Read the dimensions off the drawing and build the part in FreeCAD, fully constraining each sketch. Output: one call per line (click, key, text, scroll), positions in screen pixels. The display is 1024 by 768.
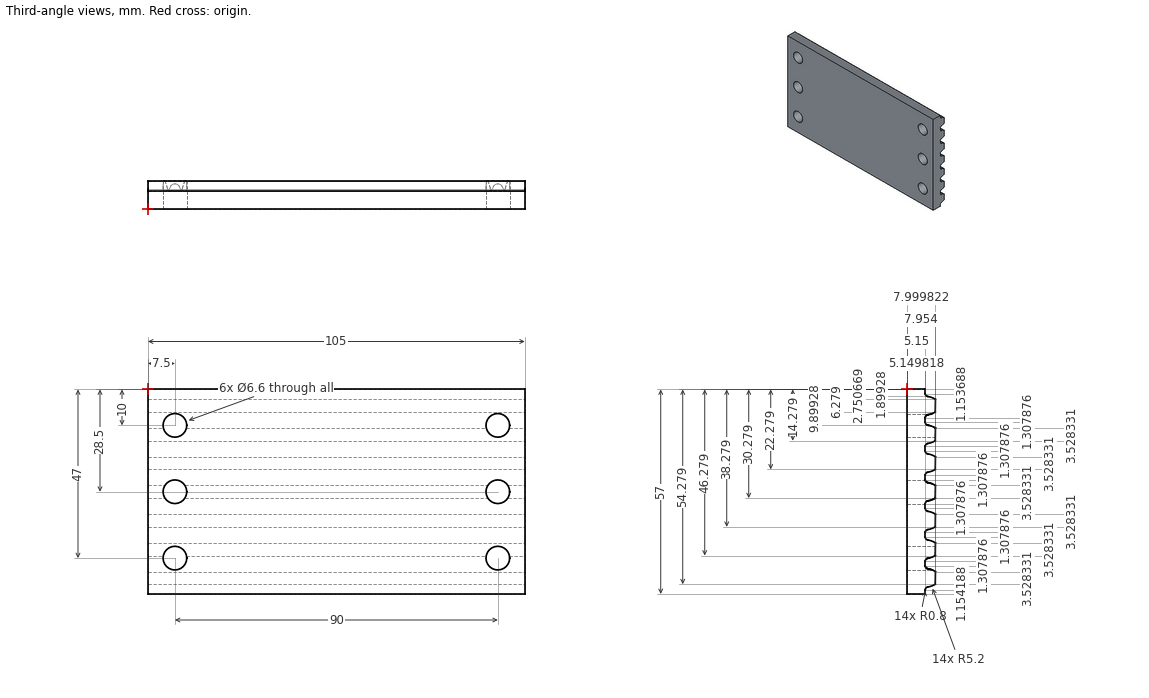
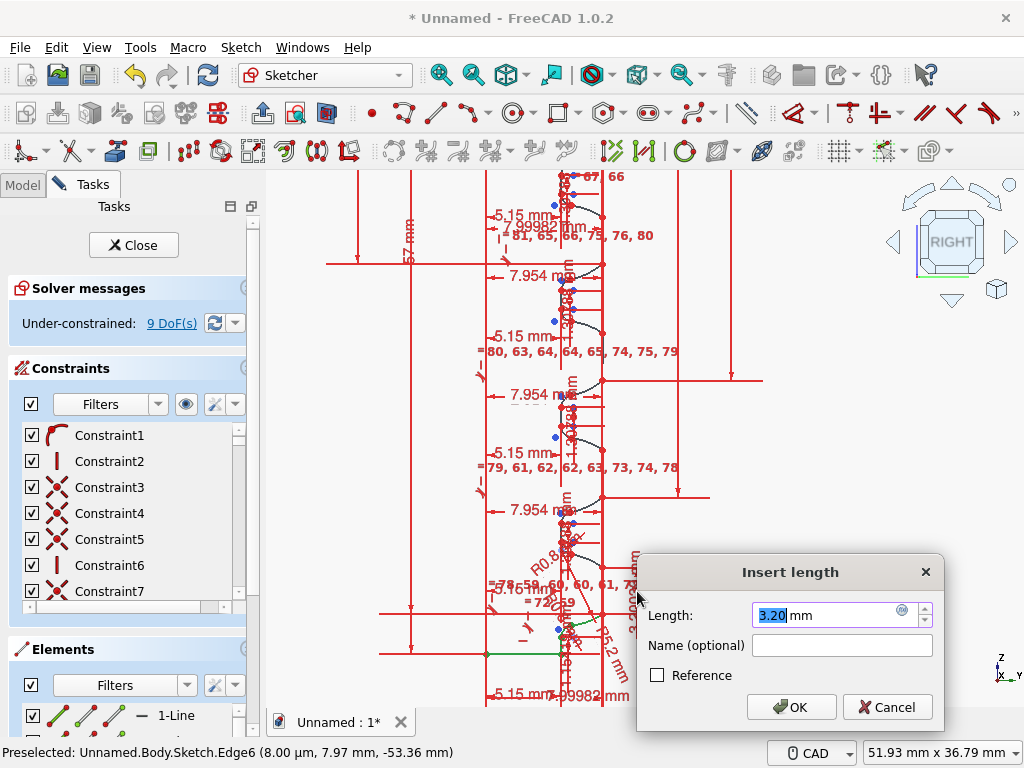
text(3.528331)
key(Return)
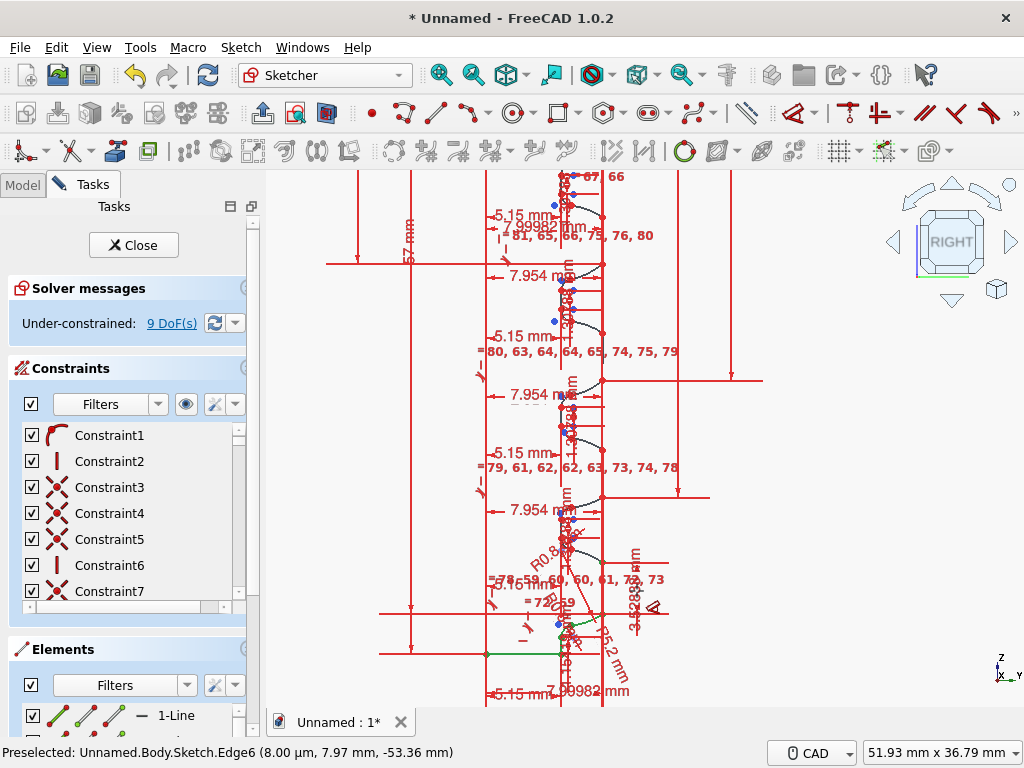
click(602, 483)
click(637, 474)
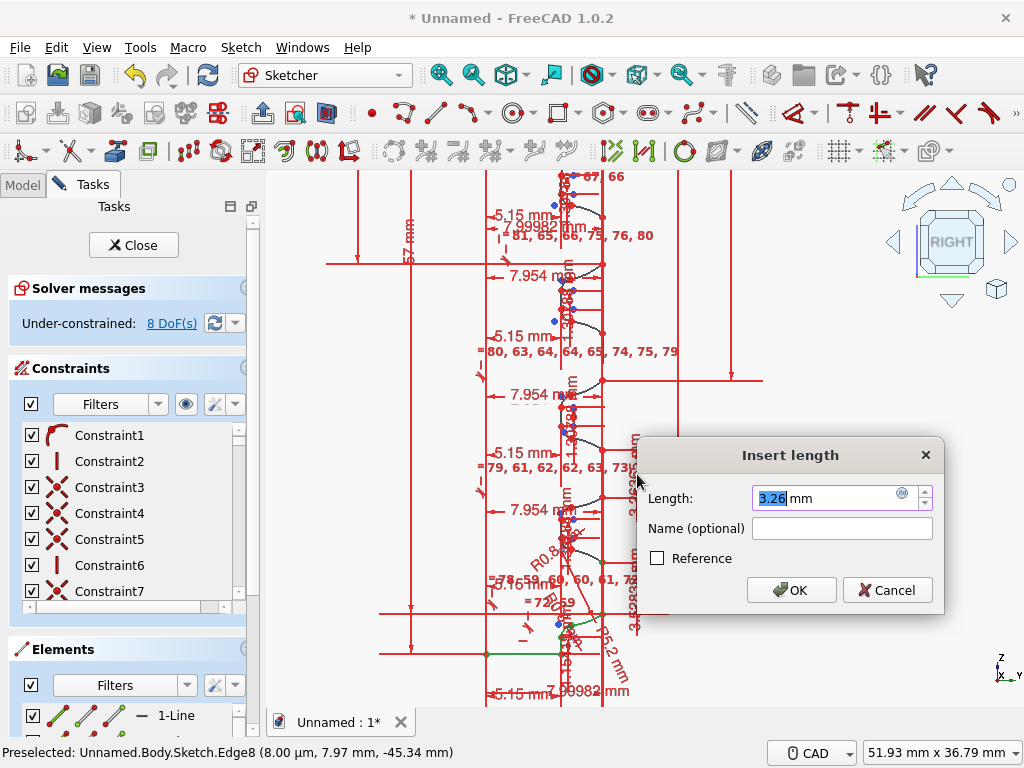
text(3.528331)
key(Return)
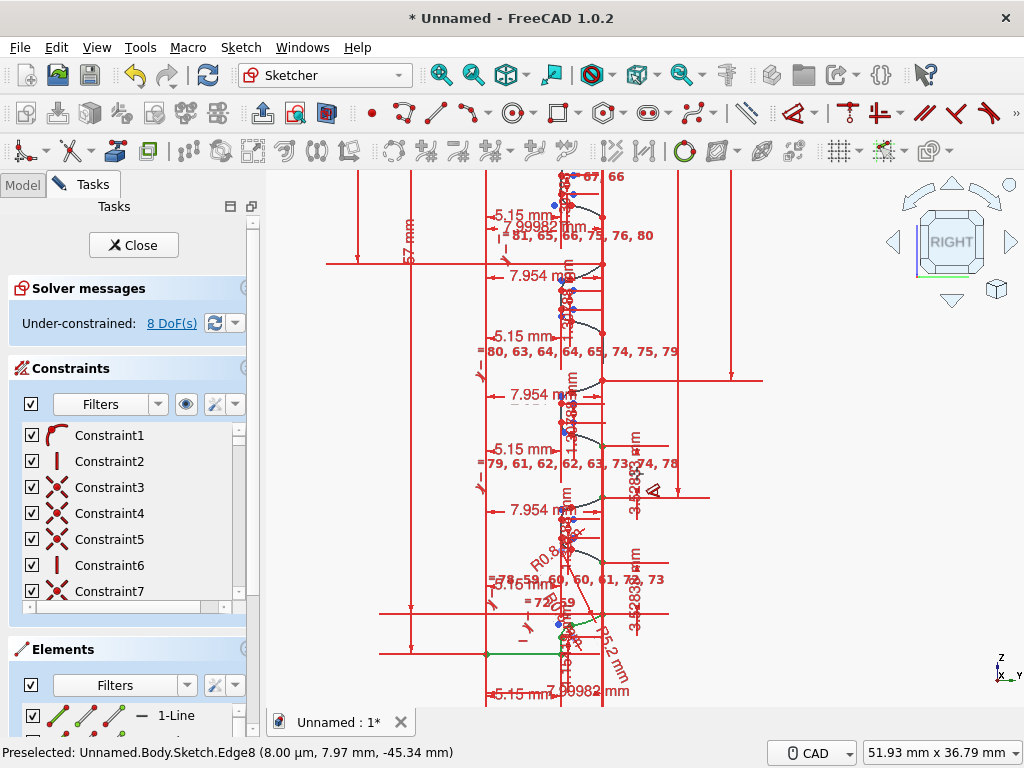
click(602, 367)
click(637, 357)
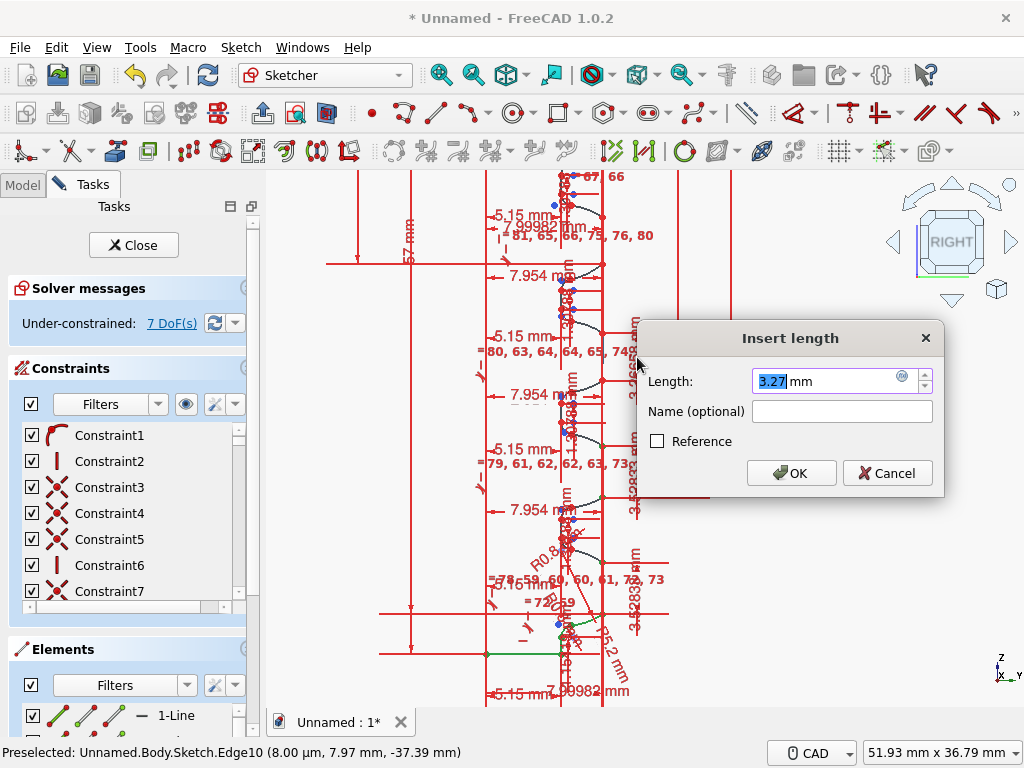
text(3.528331)
key(Return)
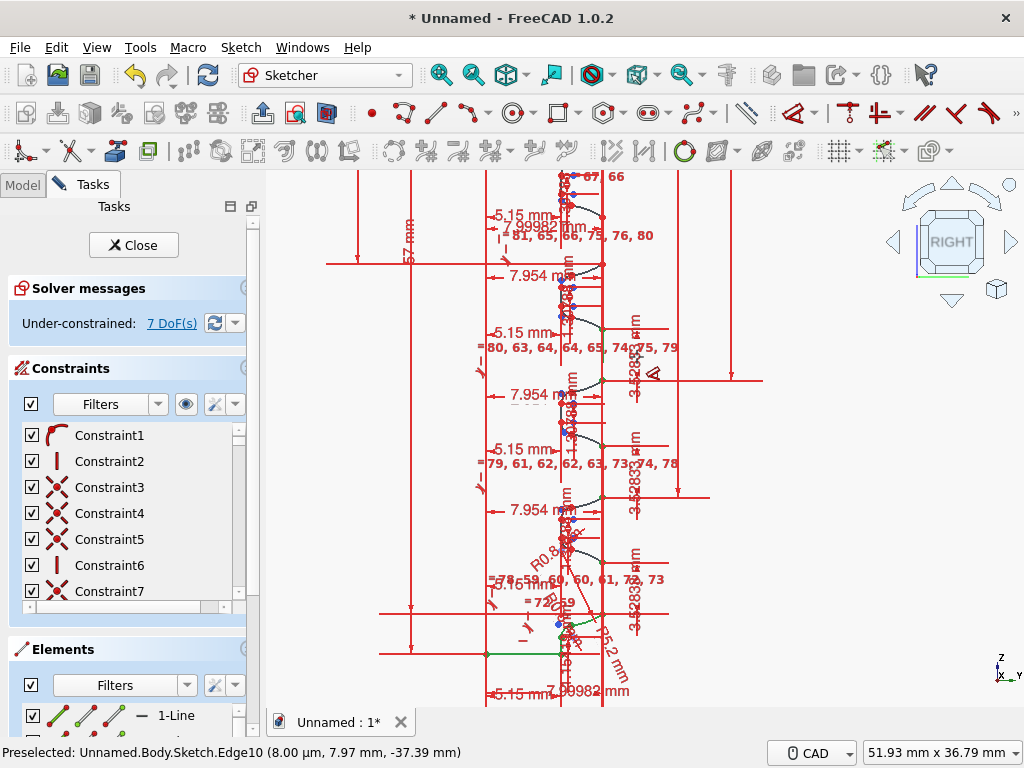
click(602, 250)
click(637, 241)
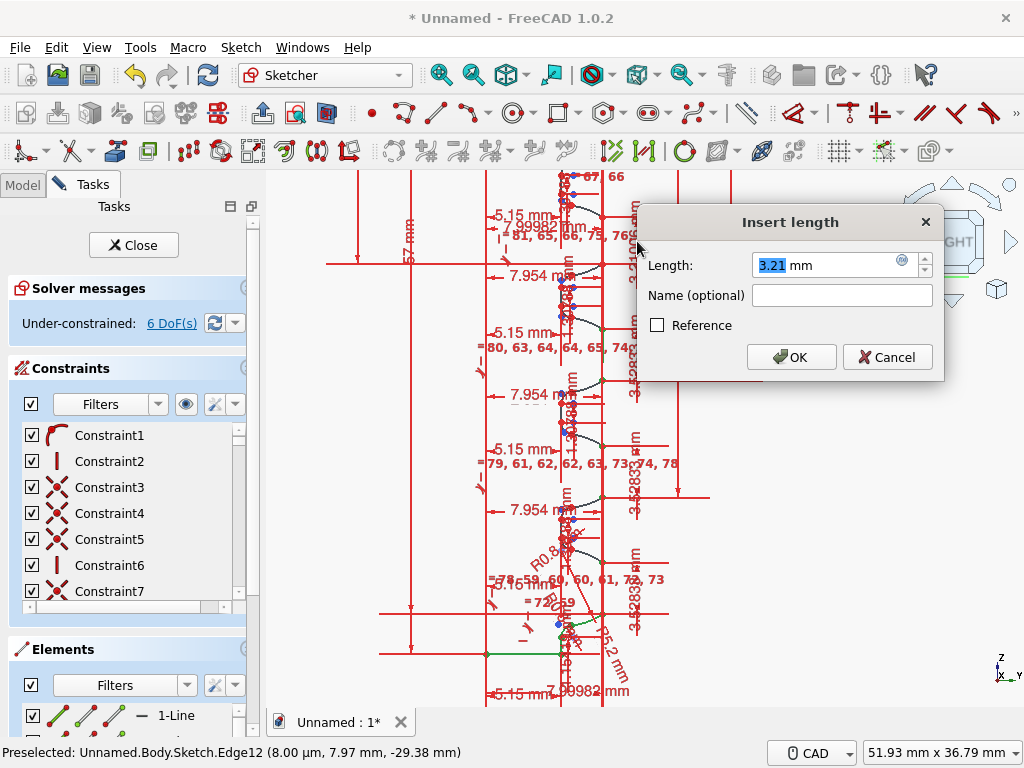
text(3.528331)
key(Return)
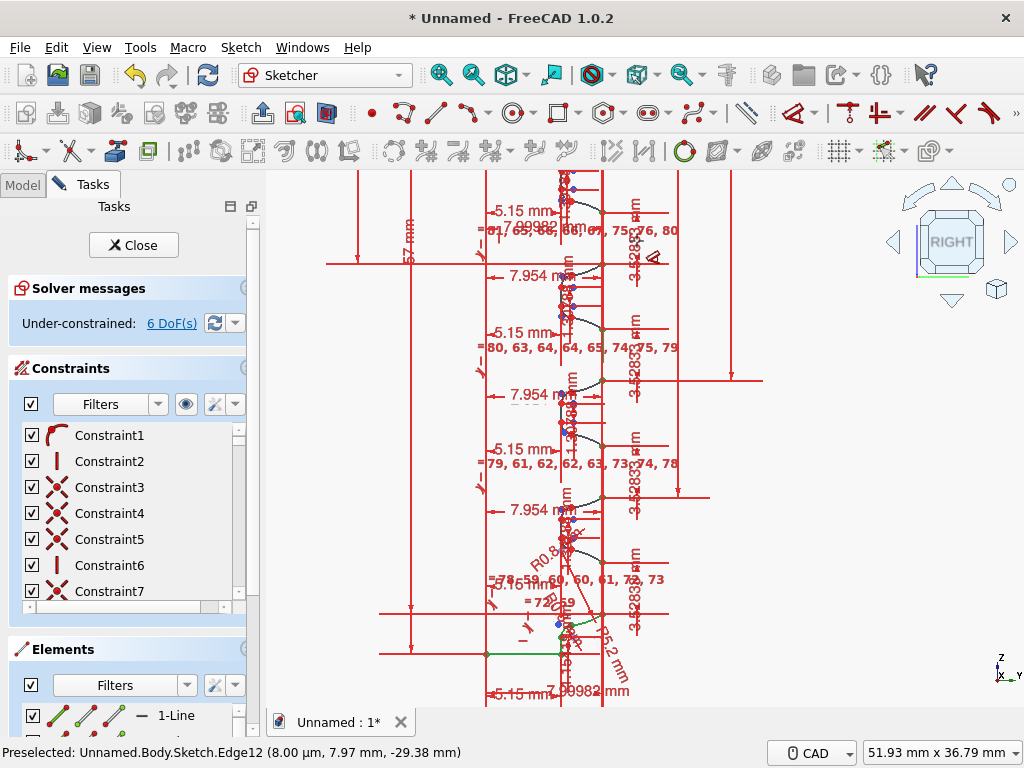
scroll(603, 602, down, 4)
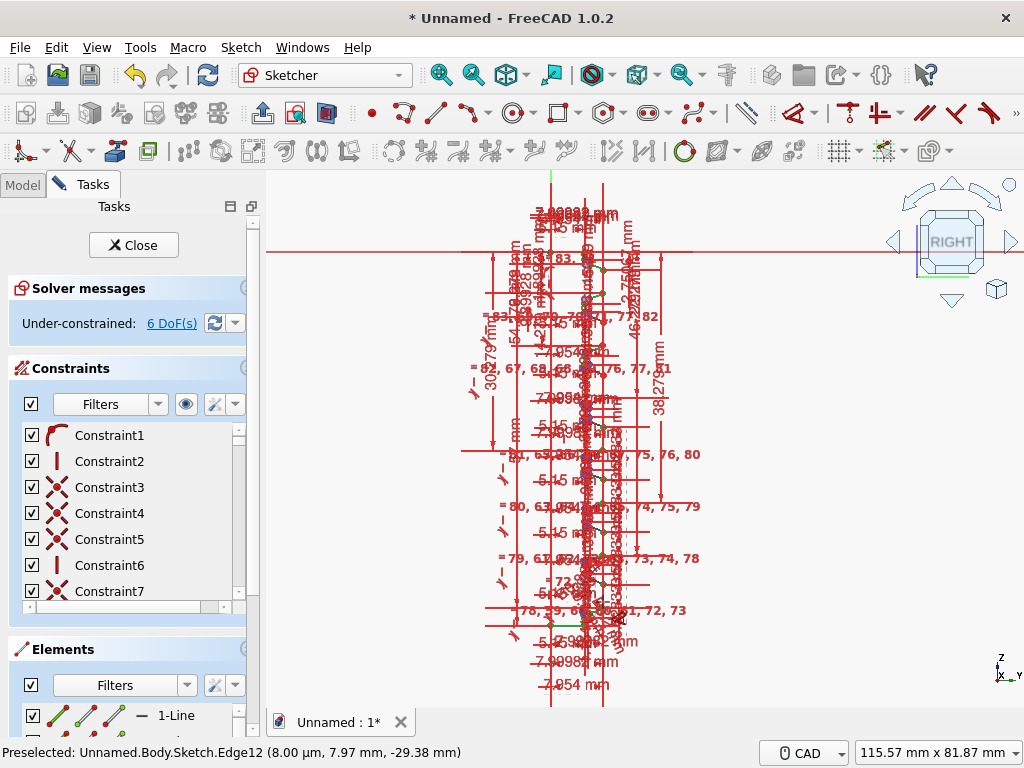
scroll(603, 391, up, 4)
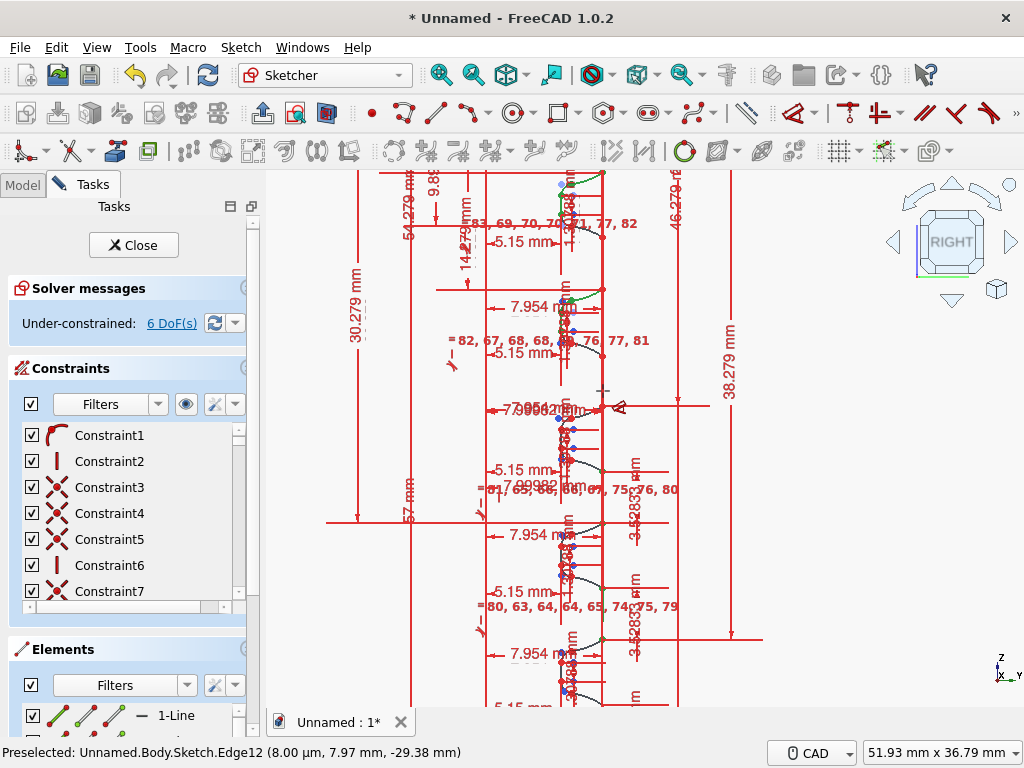
click(602, 391)
click(637, 381)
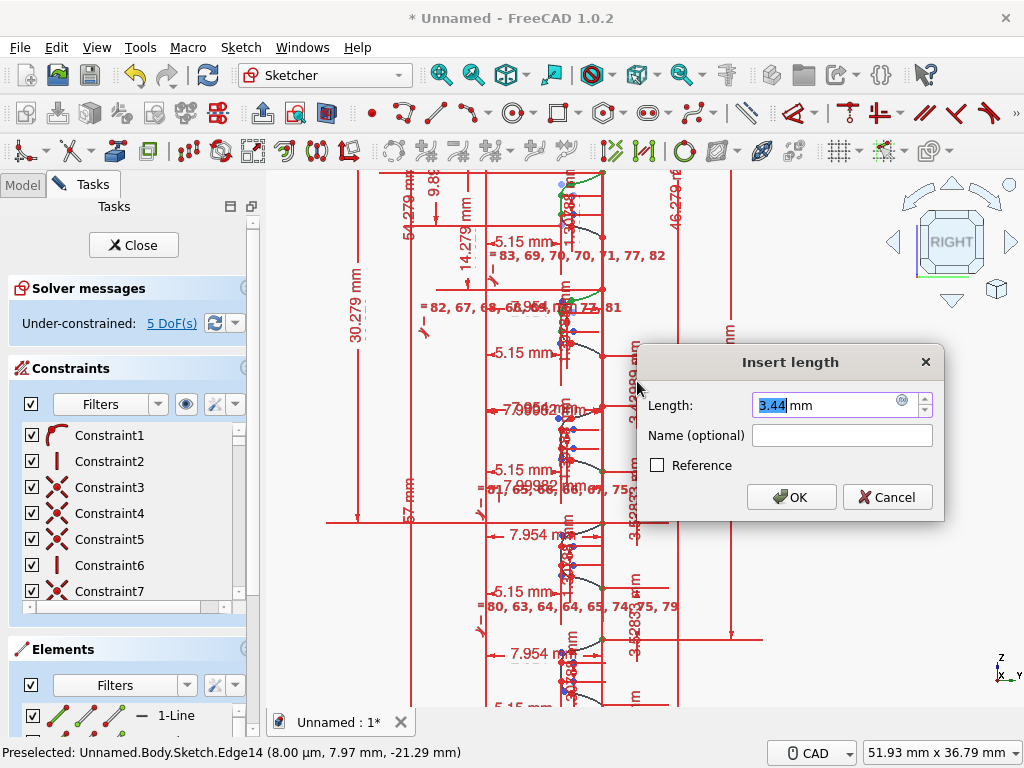
text(3.528331)
key(Return)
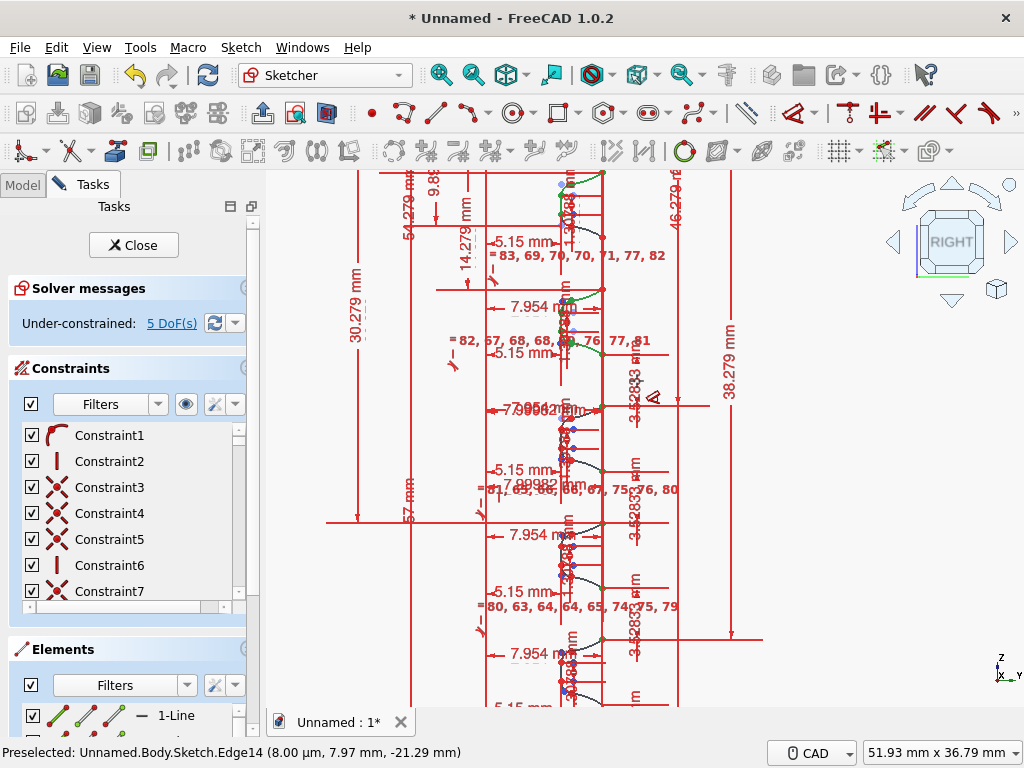
click(602, 274)
click(637, 264)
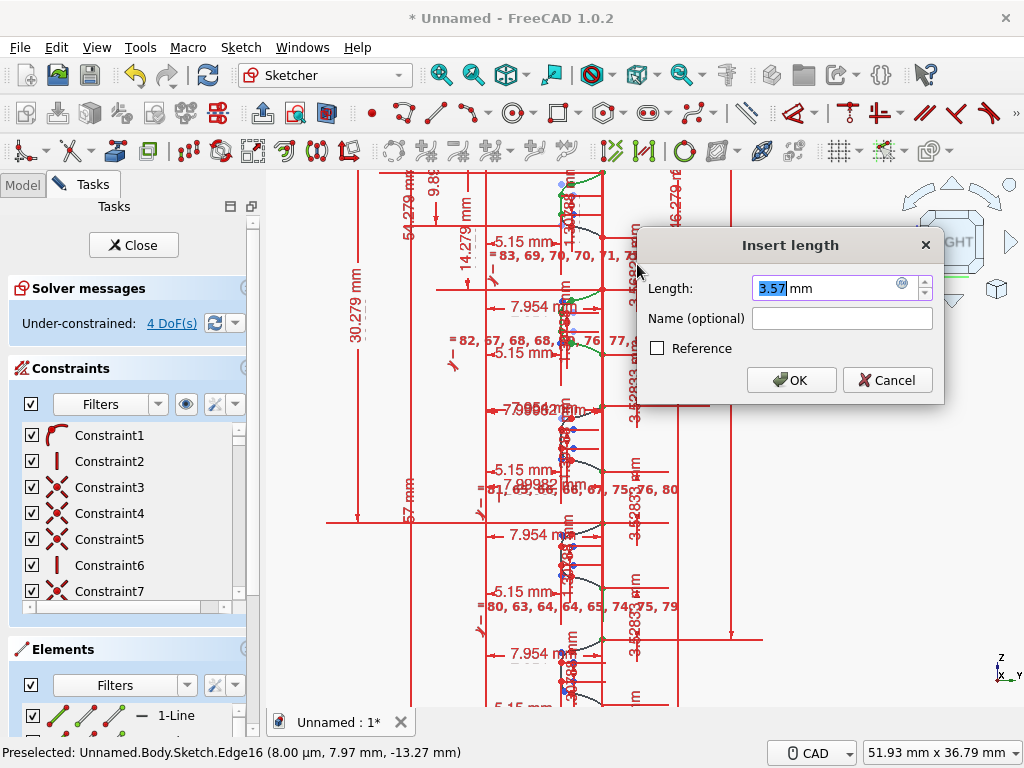
text(3.528331)
key(Return)